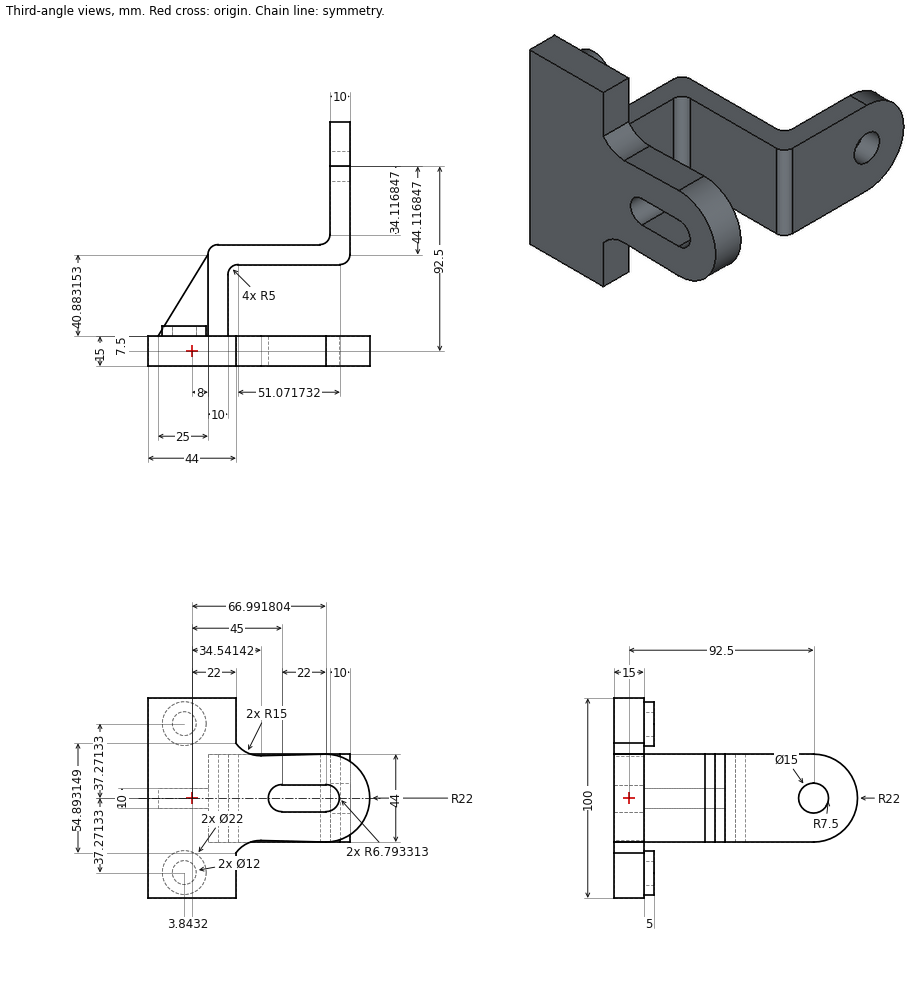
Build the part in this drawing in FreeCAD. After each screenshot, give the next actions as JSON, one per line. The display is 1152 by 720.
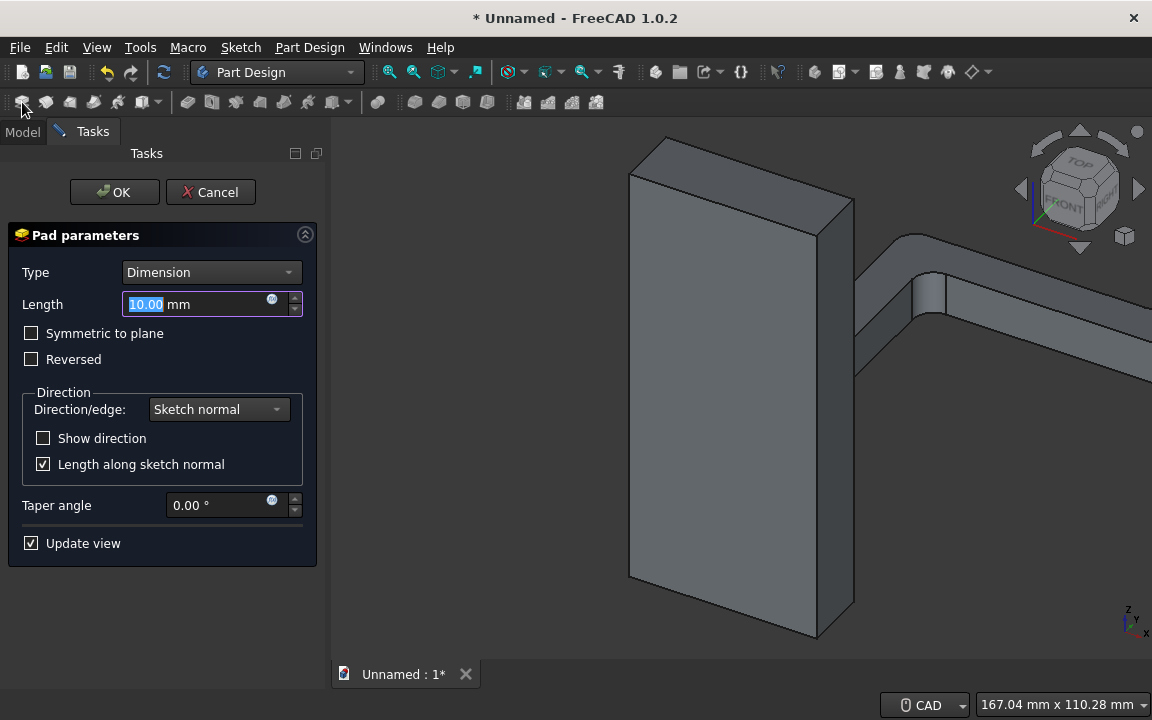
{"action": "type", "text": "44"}
{"action": "key", "text": "Tab"}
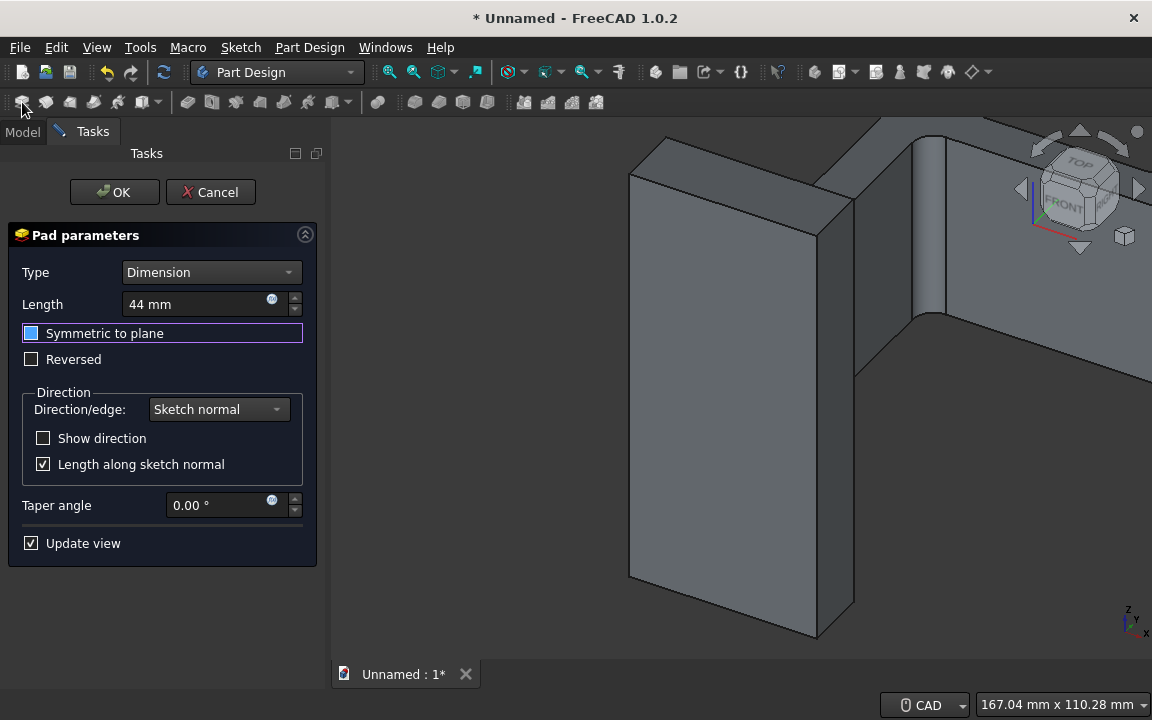
{"action": "left_click", "coordinate": [30, 333]}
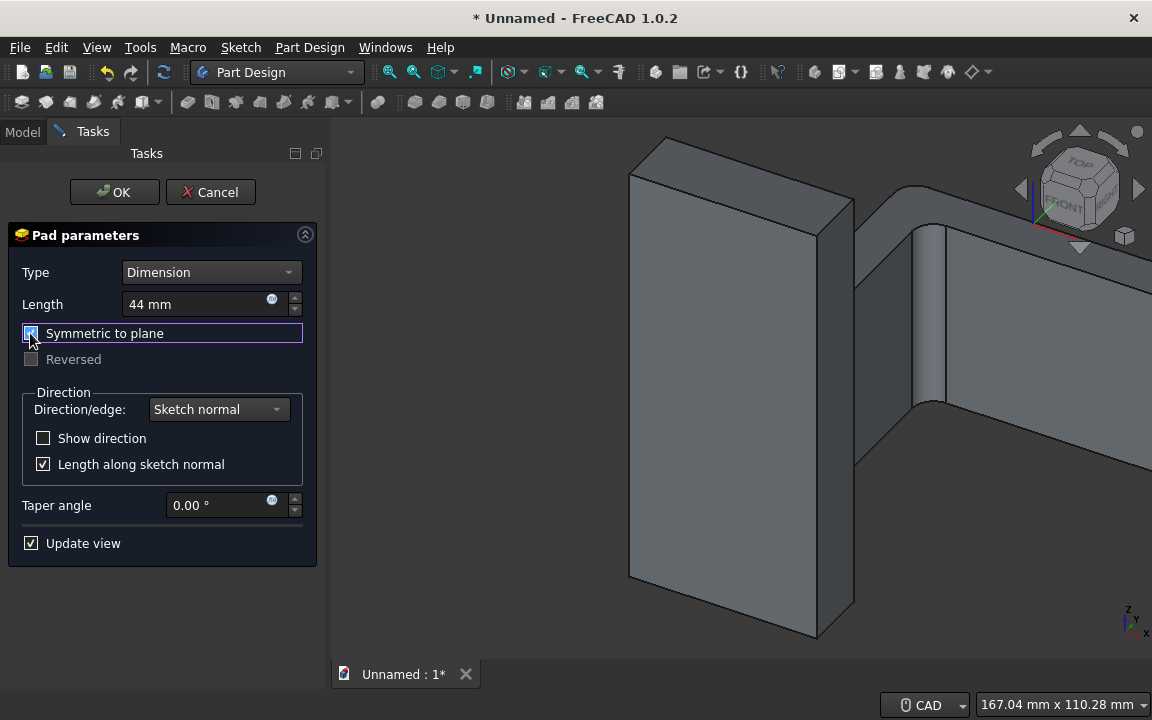
{"action": "left_click", "coordinate": [115, 192]}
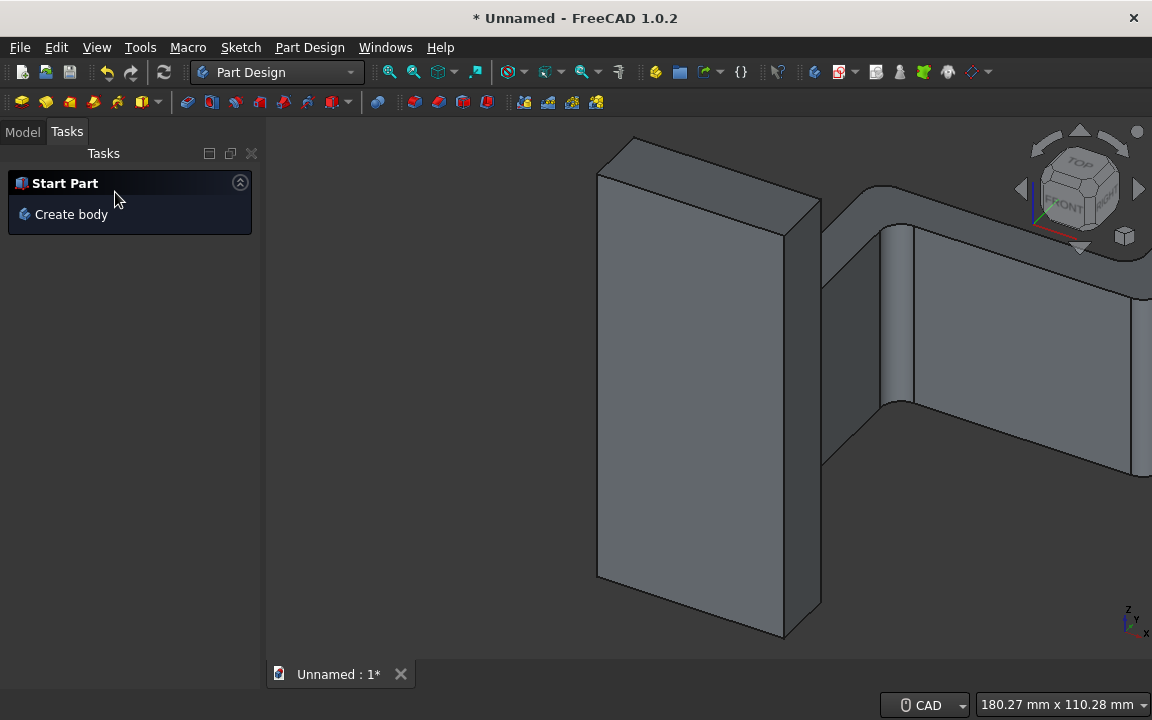
{"action": "left_click", "coordinate": [390, 72]}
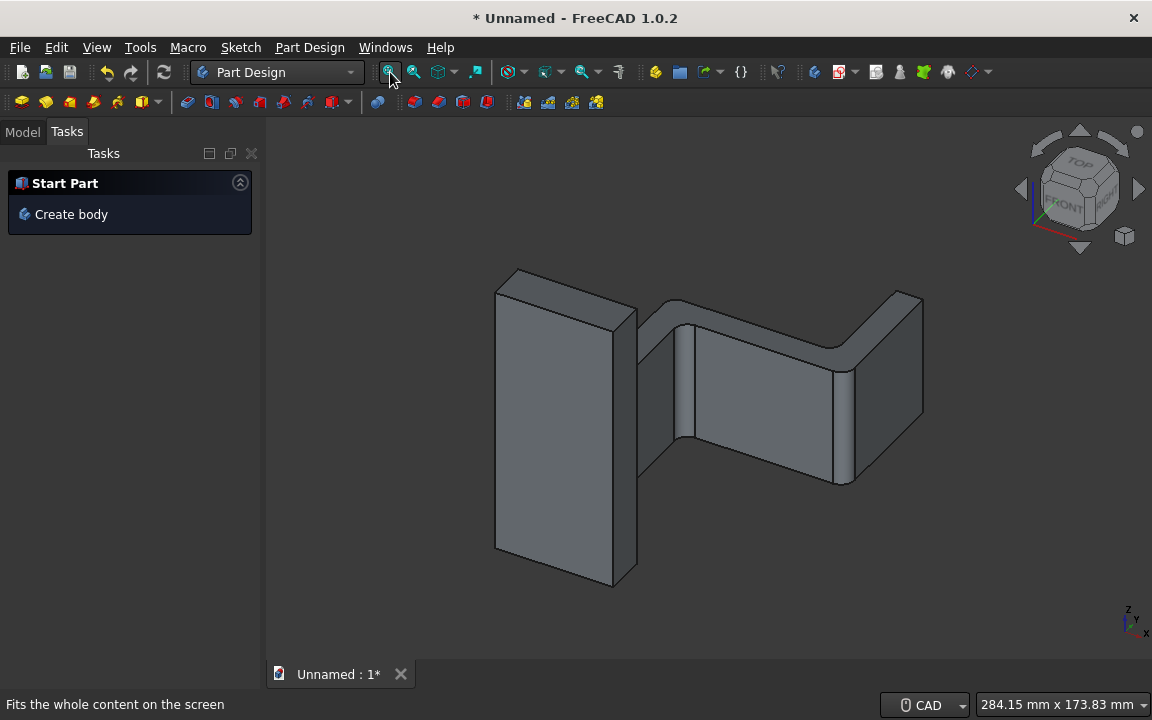
{"action": "key", "text": "6"}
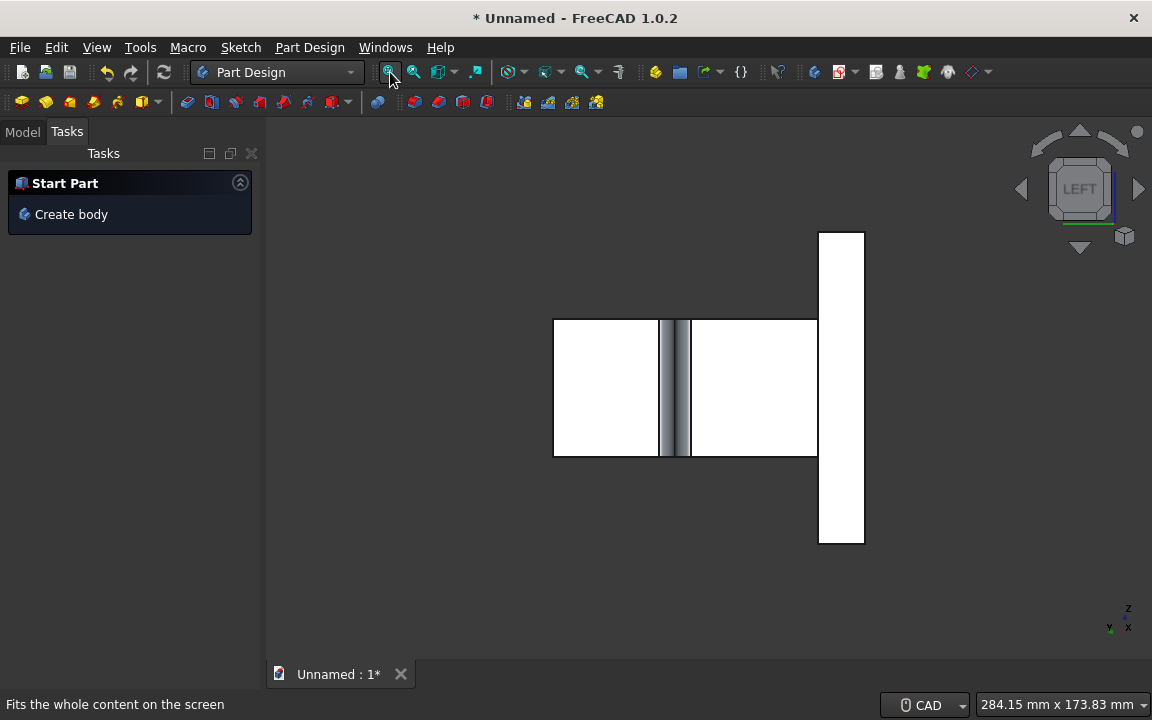
{"action": "left_click", "coordinate": [606, 387]}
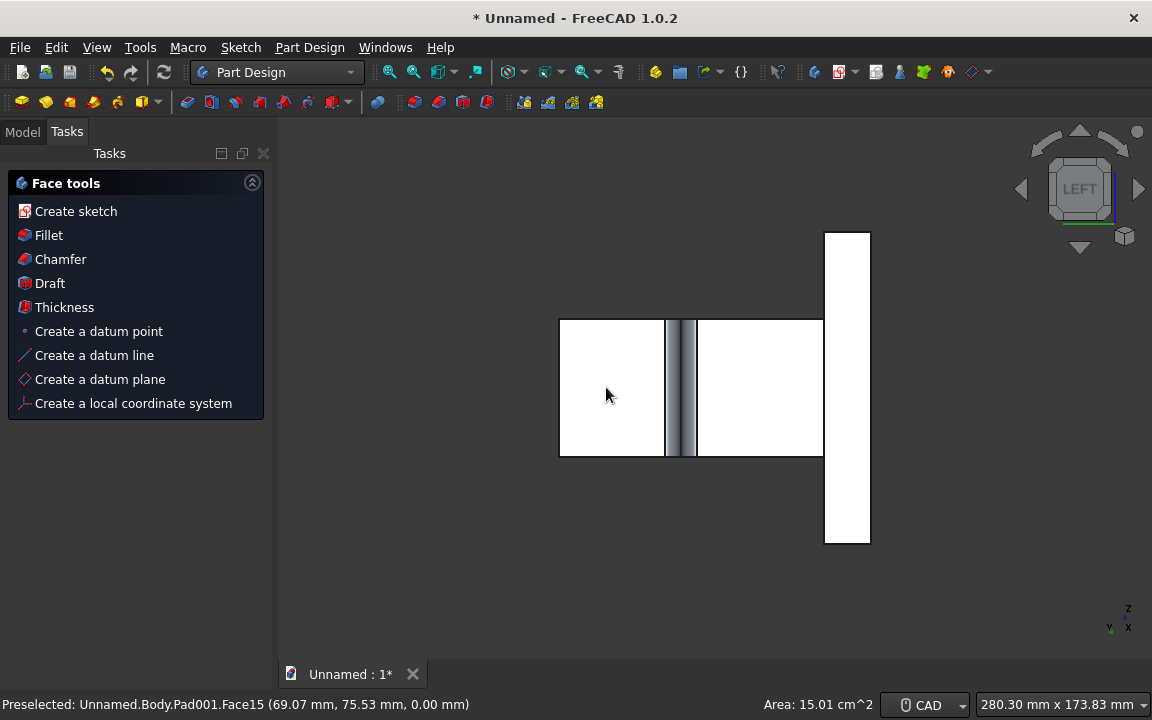
{"action": "left_click", "coordinate": [840, 72]}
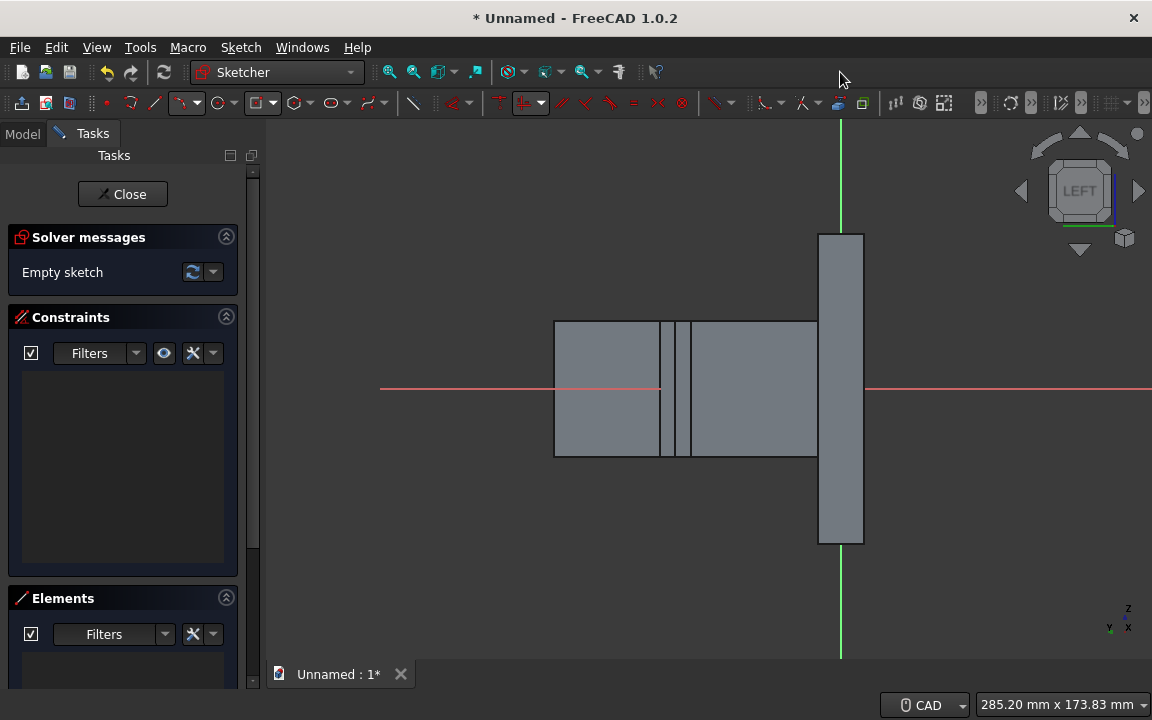
{"action": "left_click", "coordinate": [70, 104]}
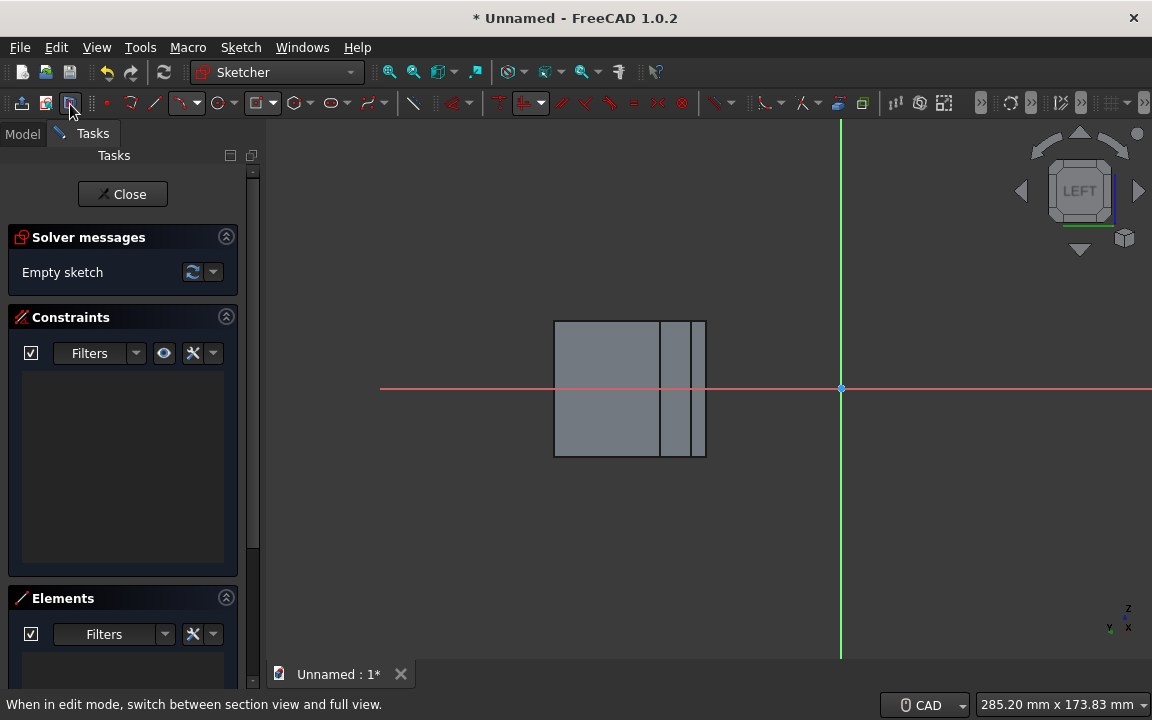
{"action": "scroll", "coordinate": [449, 389], "scroll_direction": "up", "scroll_amount": 5}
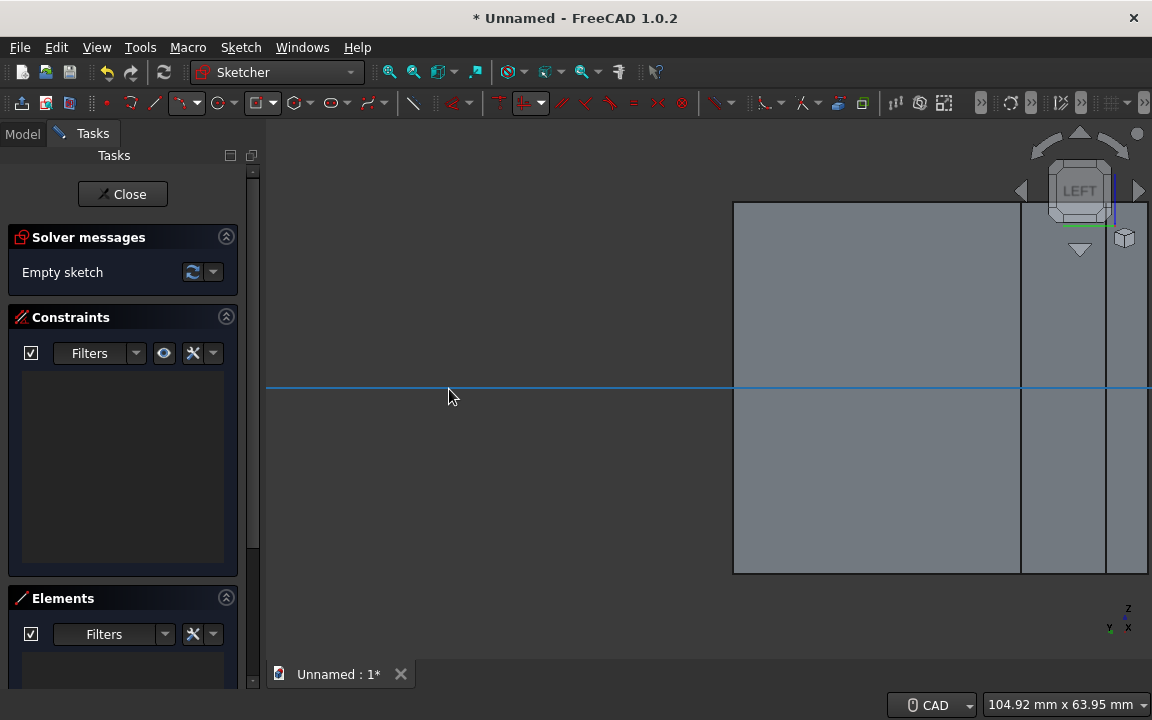
{"action": "left_click", "coordinate": [156, 104]}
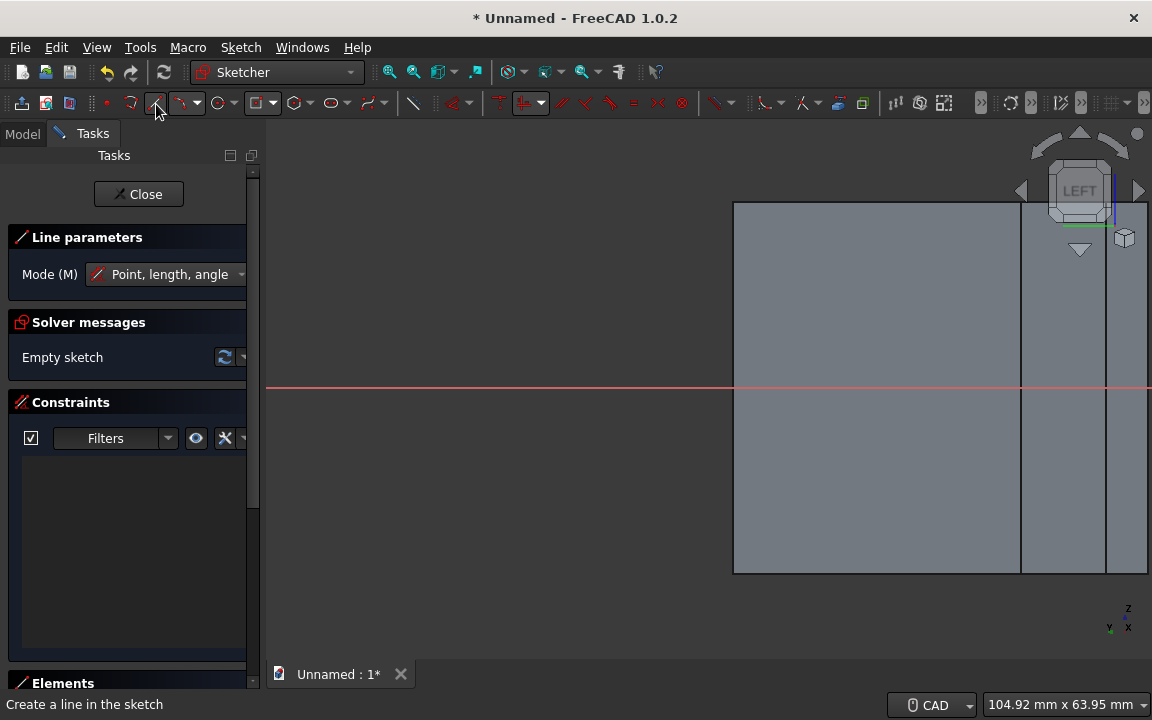
{"action": "left_click", "coordinate": [733, 325]}
{"action": "left_click", "coordinate": [733, 202]}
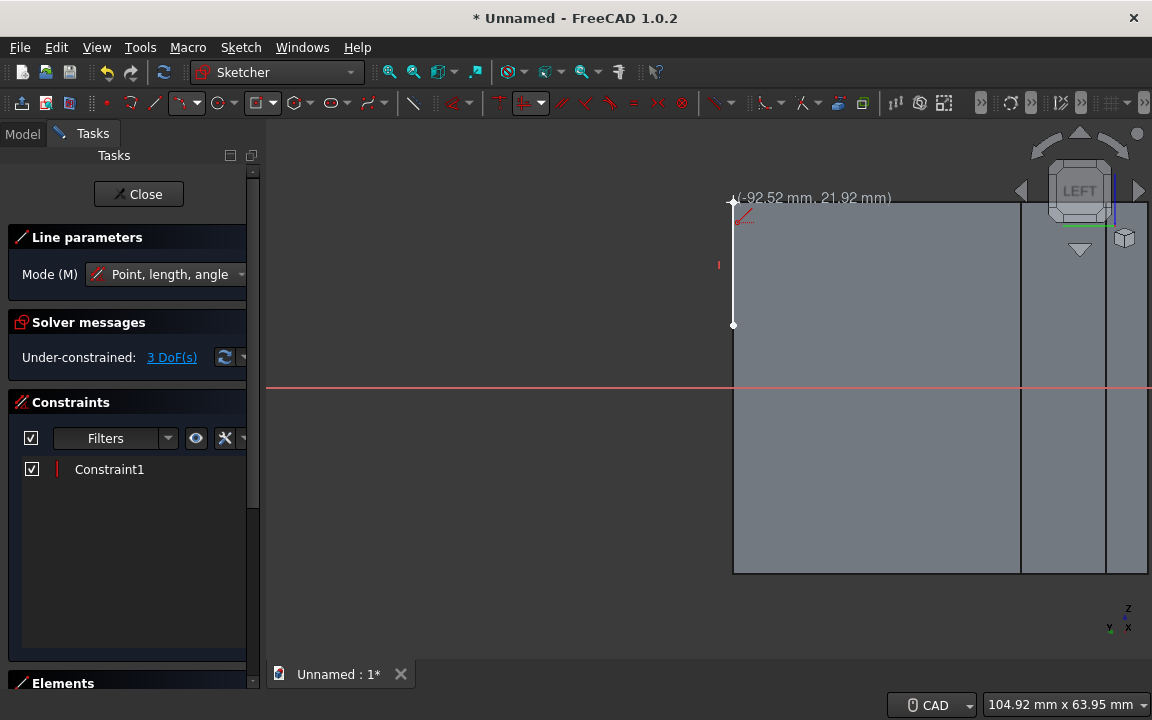
{"action": "left_click", "coordinate": [733, 574]}
{"action": "left_click", "coordinate": [733, 451]}